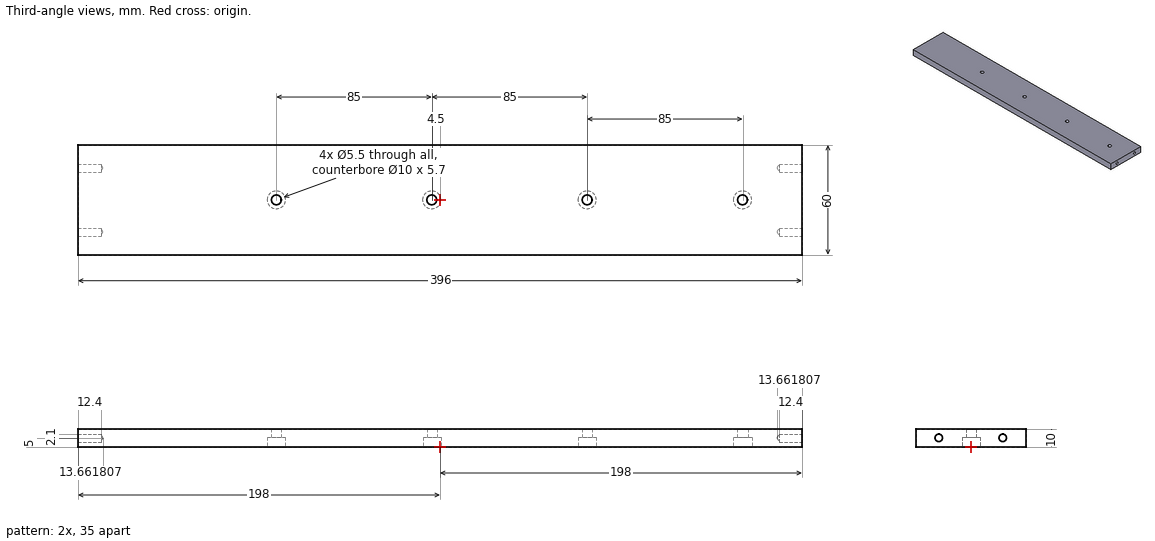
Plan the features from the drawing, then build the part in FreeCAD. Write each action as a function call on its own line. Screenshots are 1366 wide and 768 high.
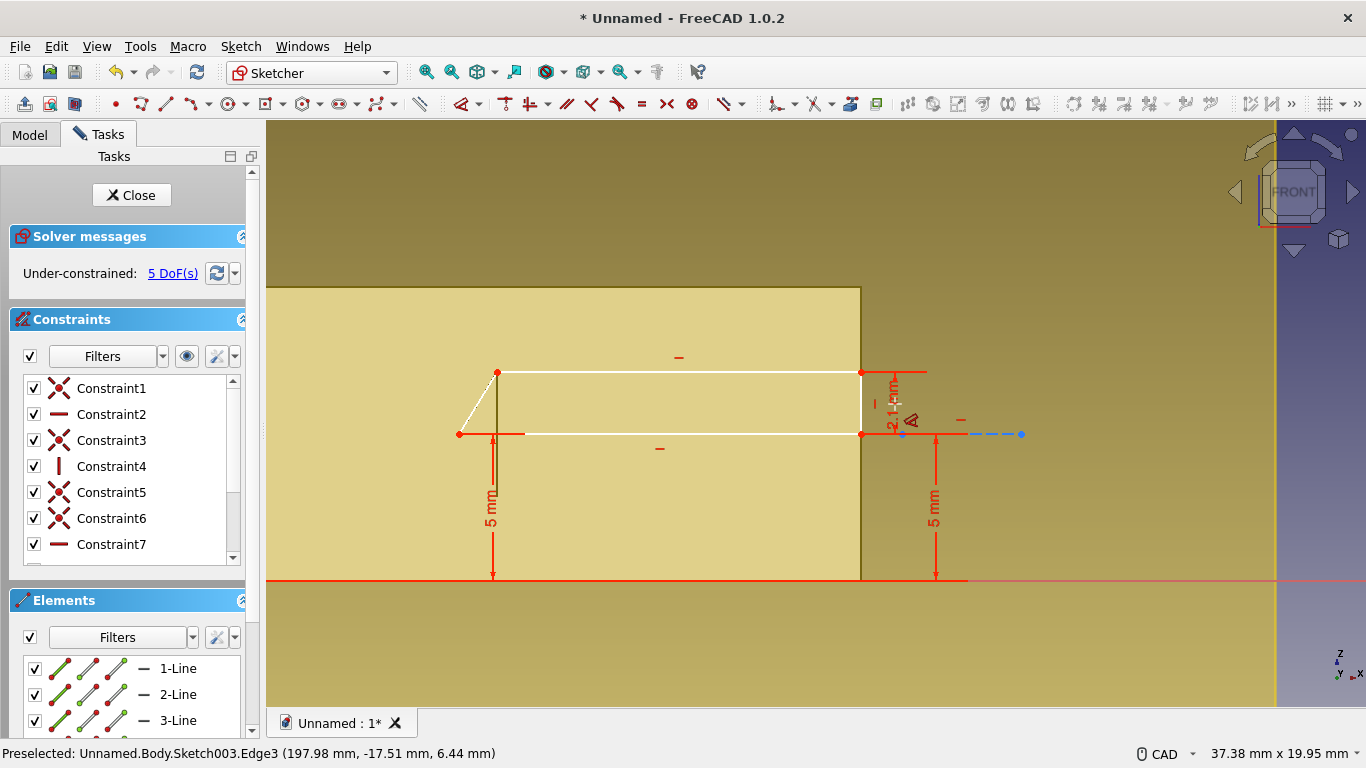
click(606, 372)
click(679, 338)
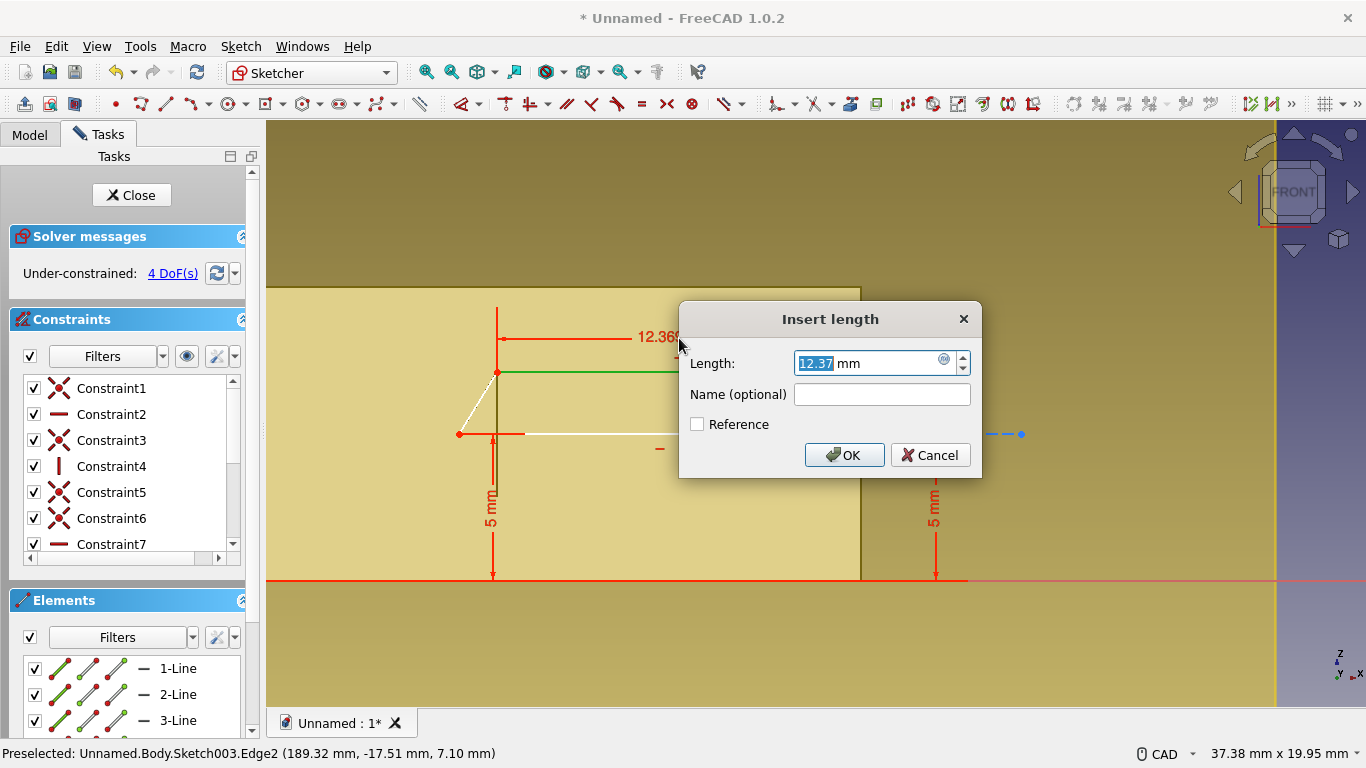
text(12.4)
key(Return)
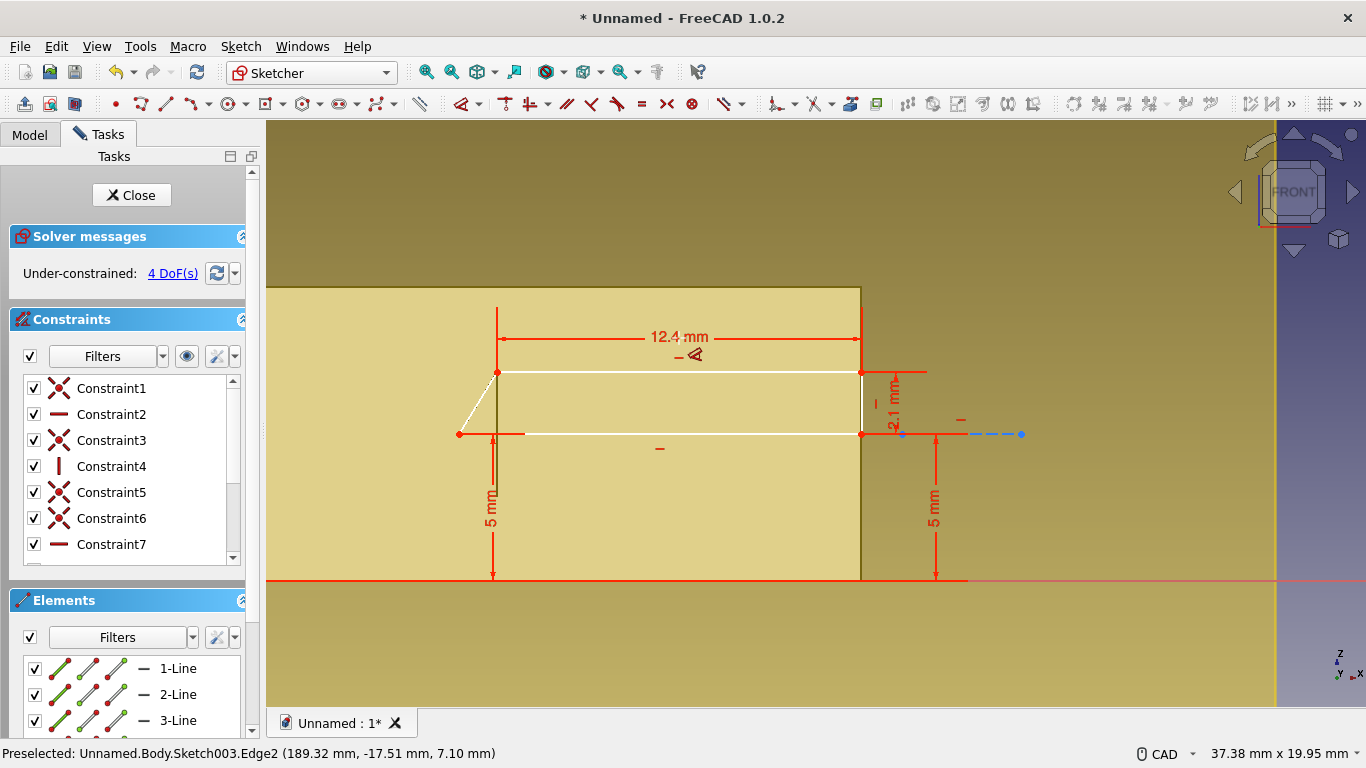
click(862, 372)
click(578, 615)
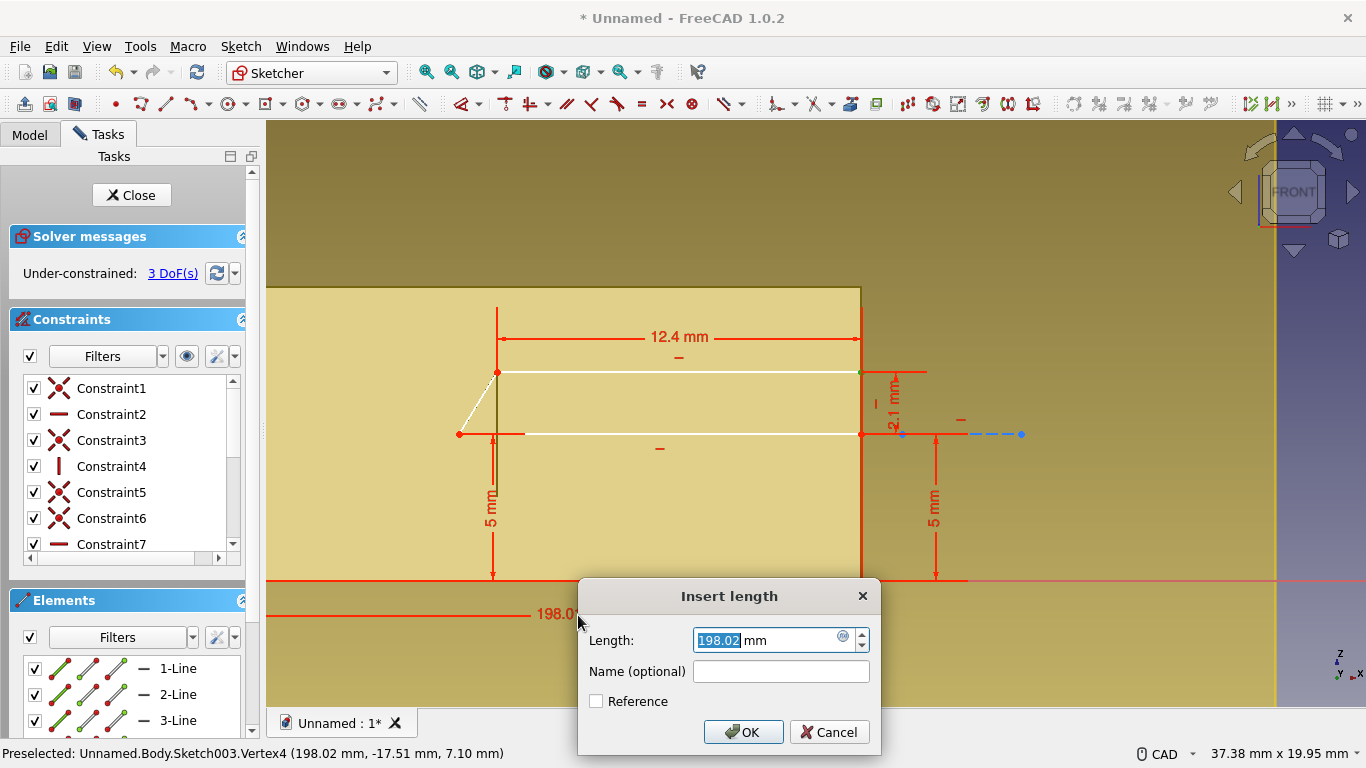
text(198)
key(Return)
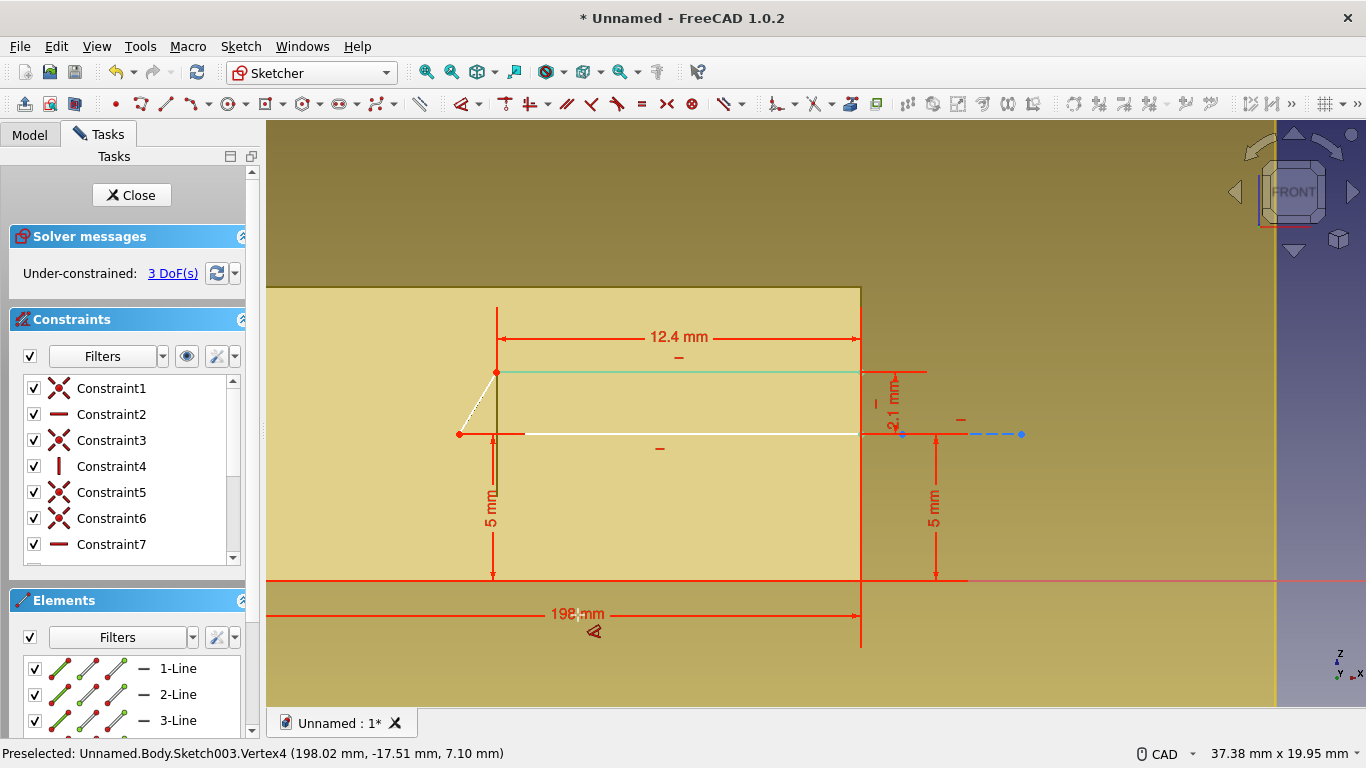
click(741, 434)
click(660, 468)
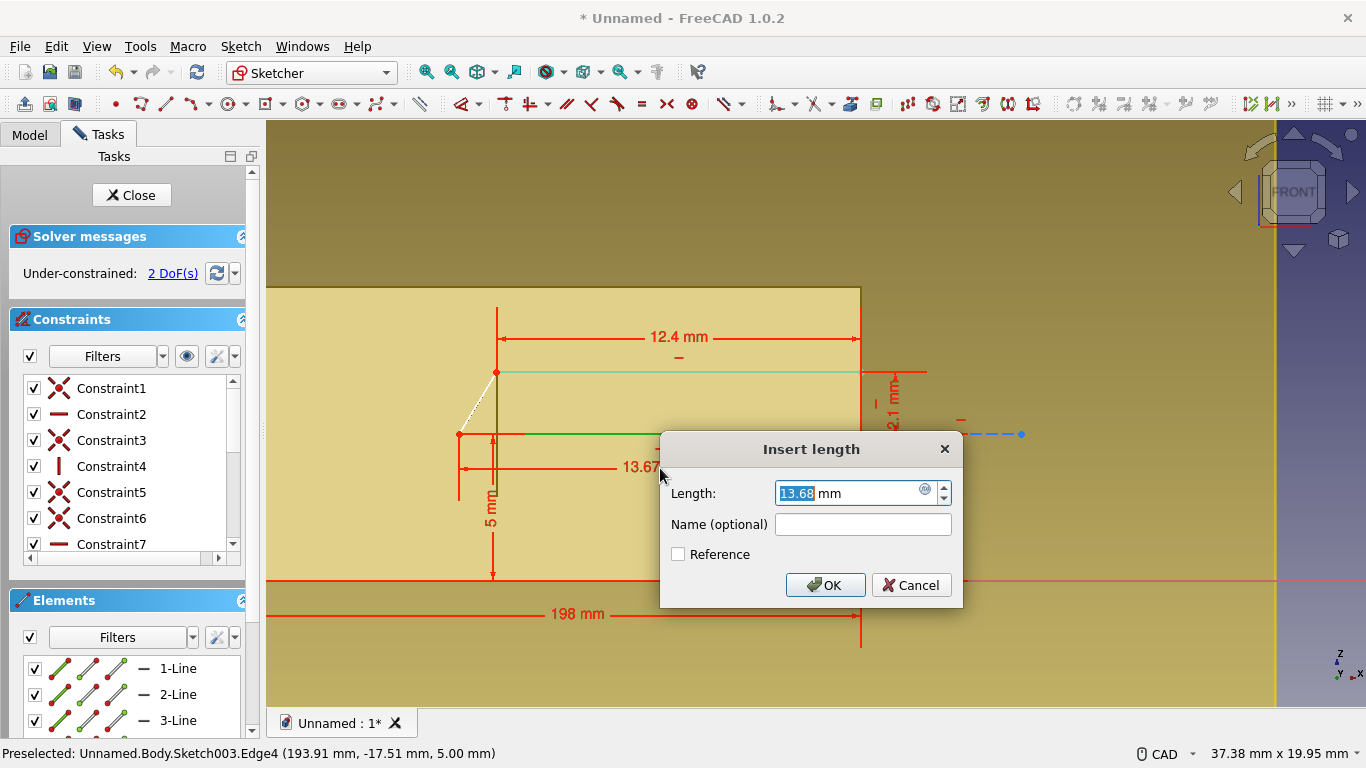
text(13.661807)
key(Return)
key(Escape)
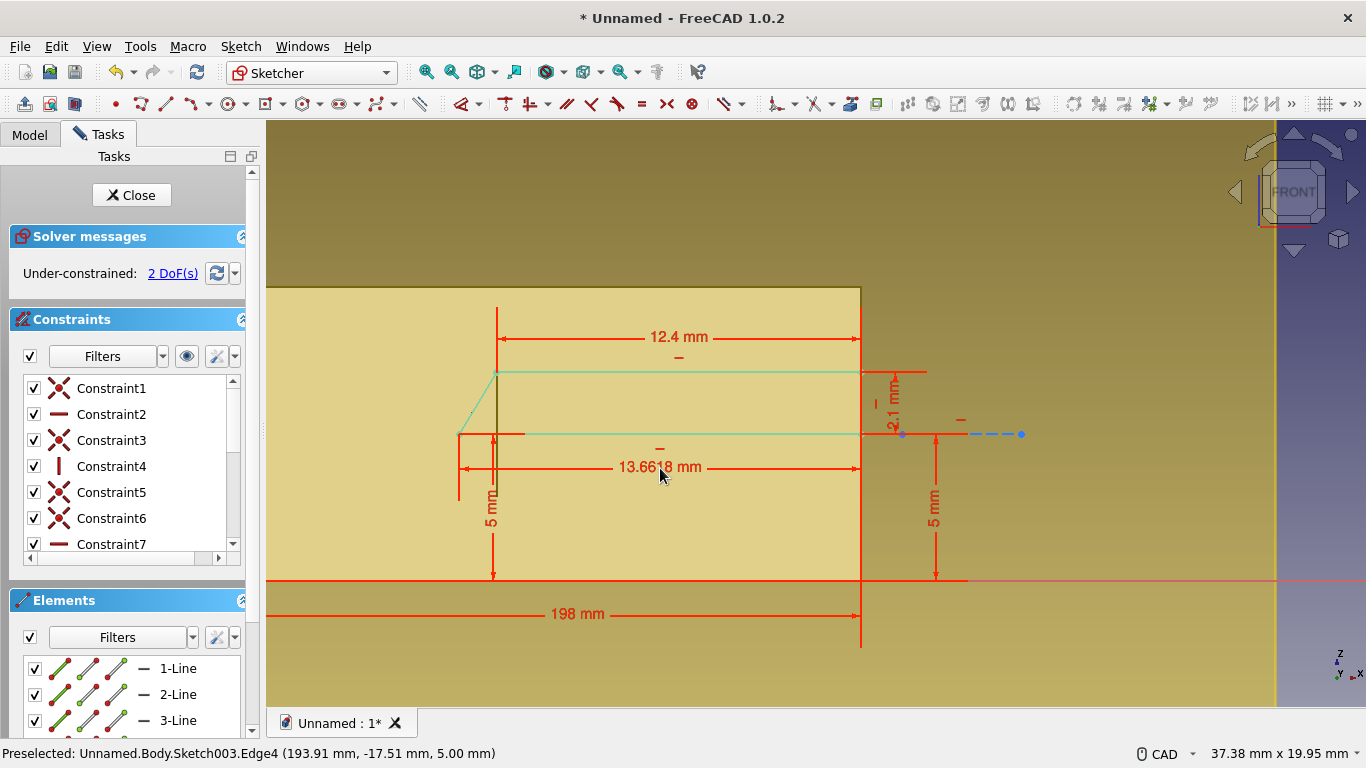
click(132, 195)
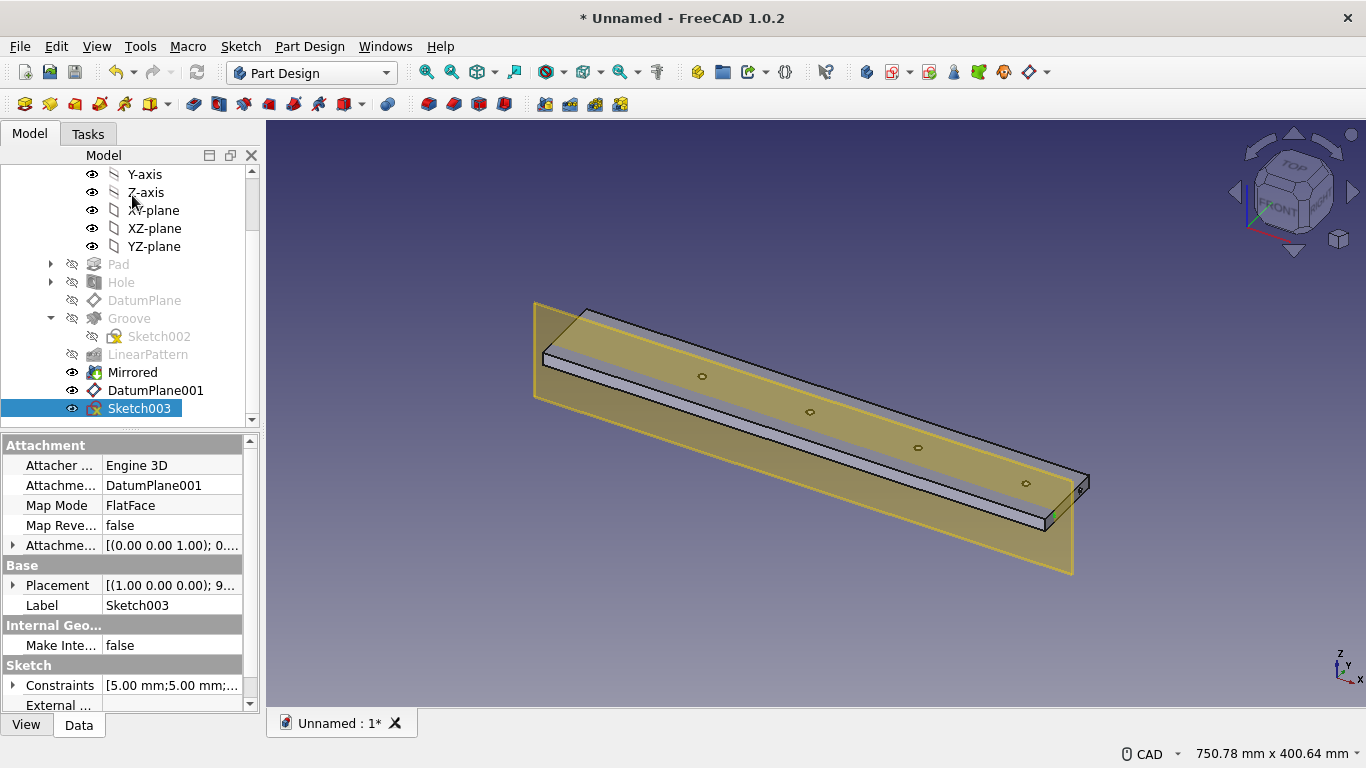
click(244, 104)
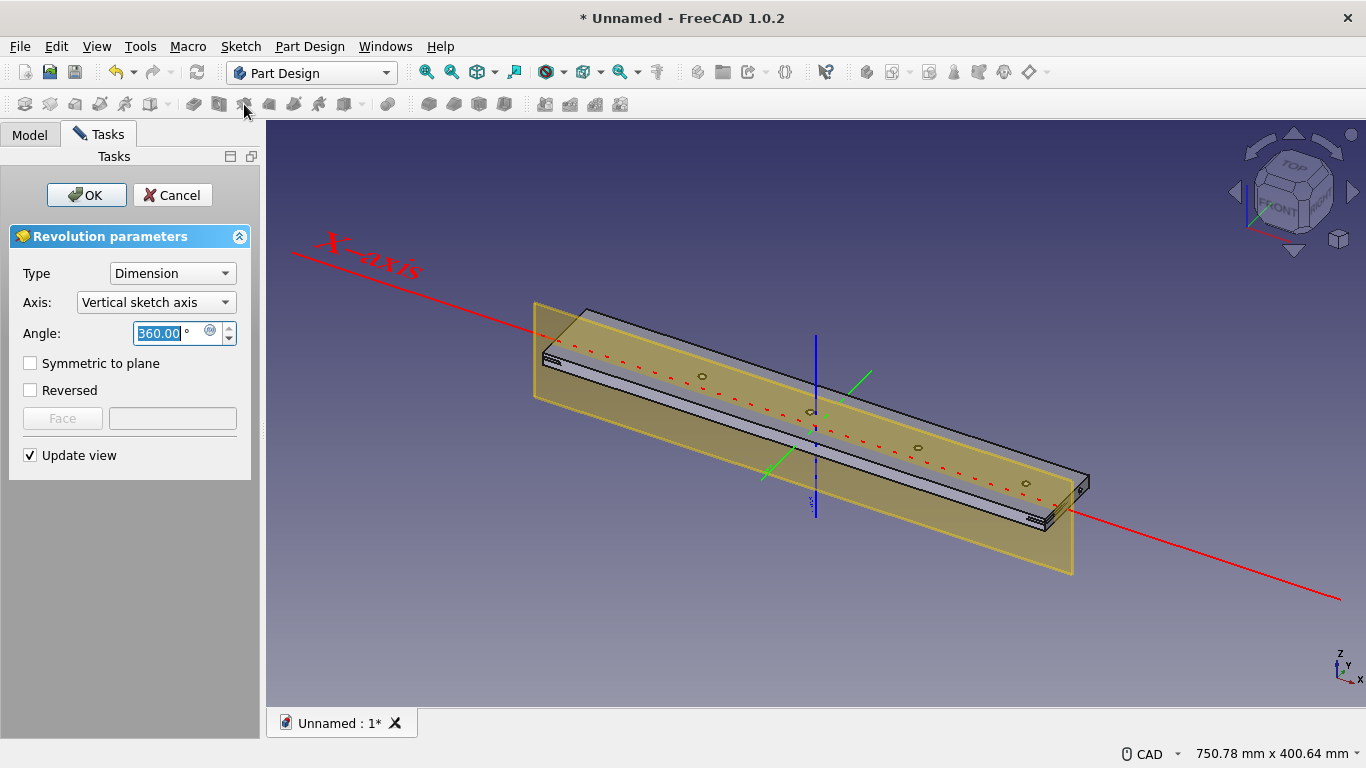
click(157, 302)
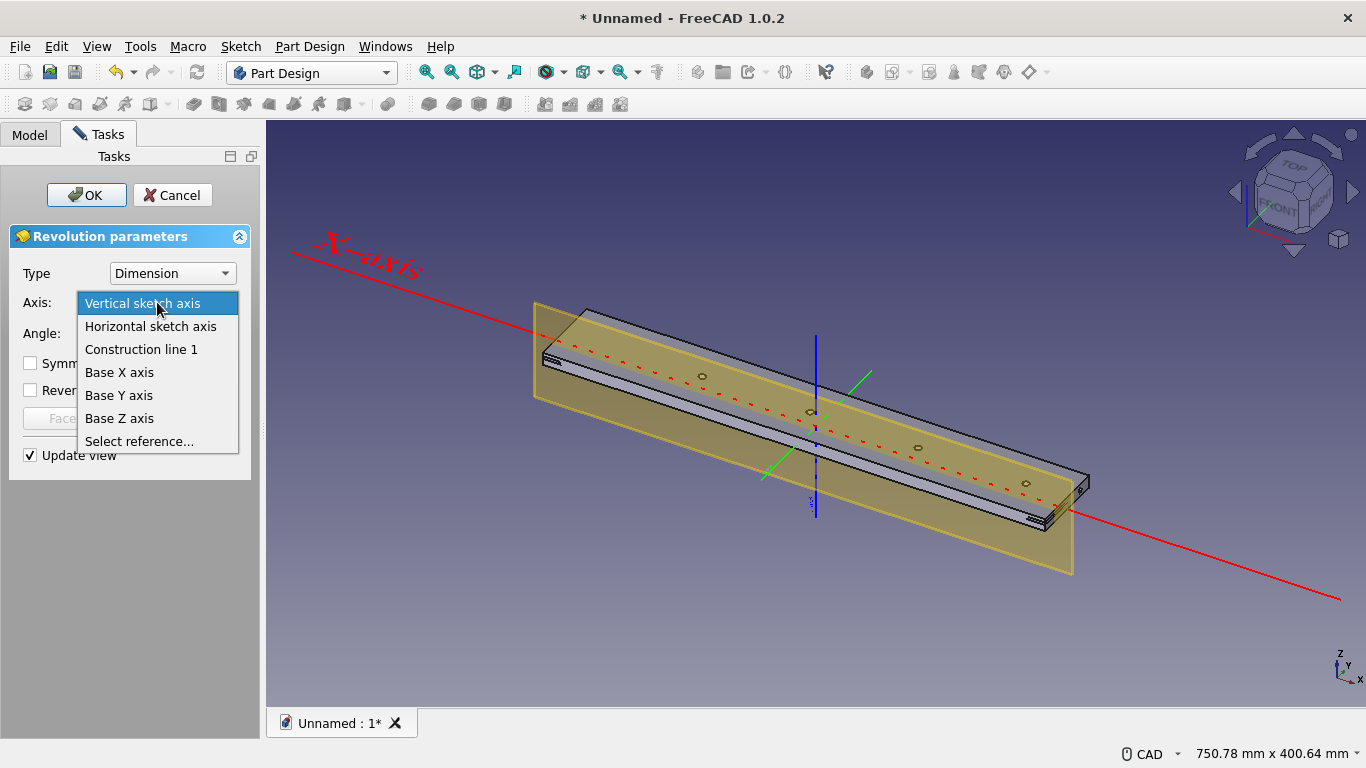
click(156, 350)